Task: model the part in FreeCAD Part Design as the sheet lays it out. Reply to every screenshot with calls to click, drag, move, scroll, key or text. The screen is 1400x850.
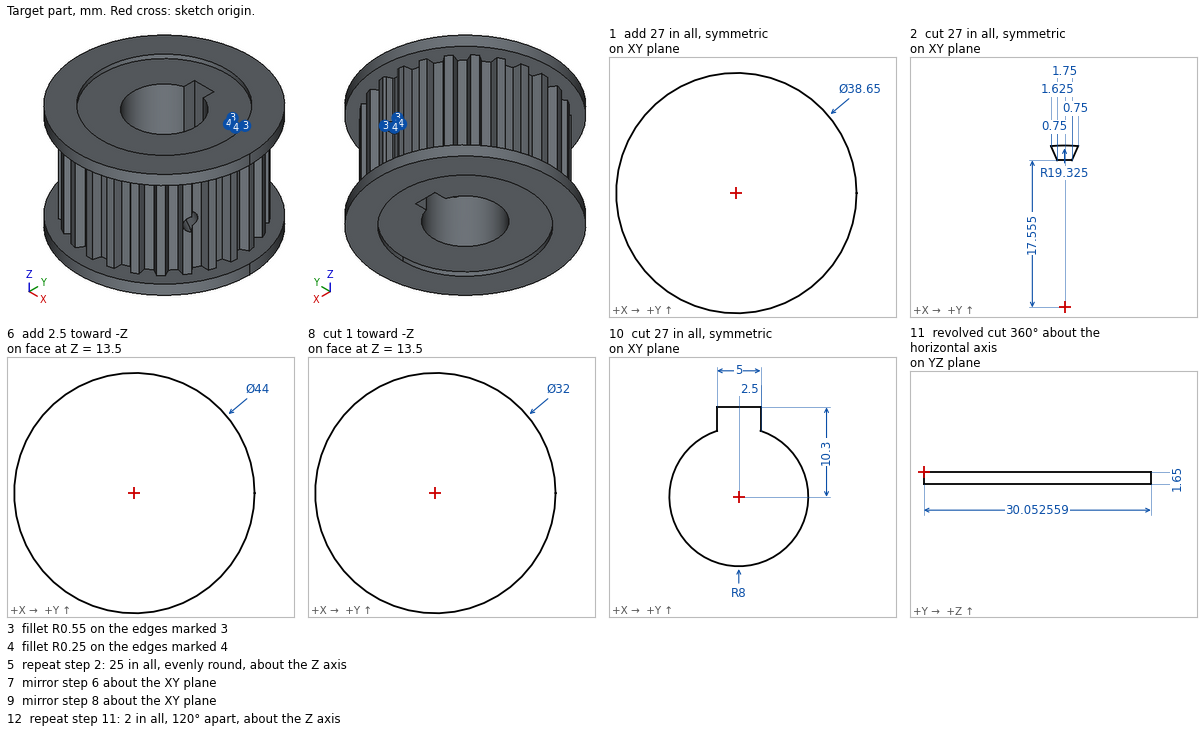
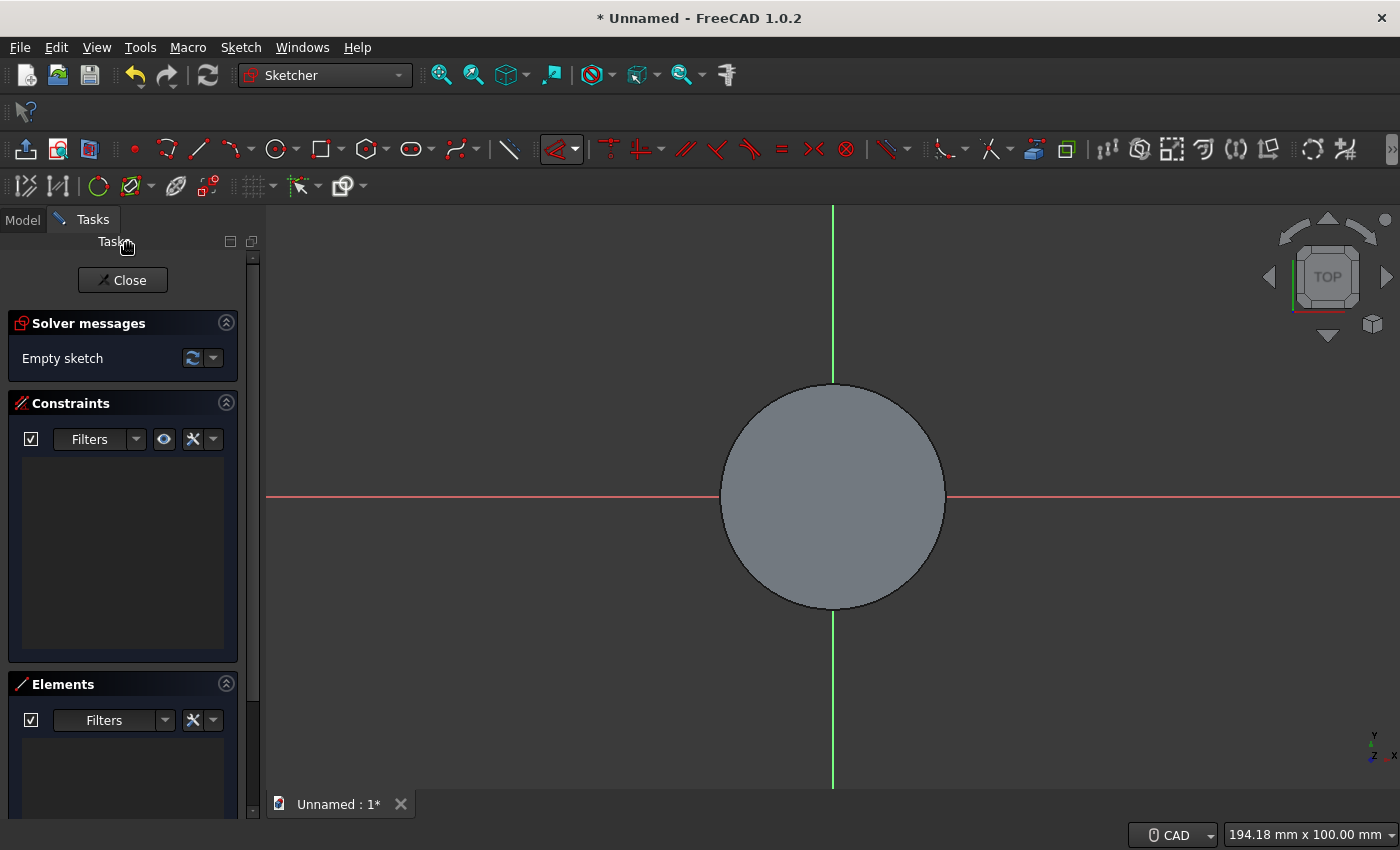
click(90, 150)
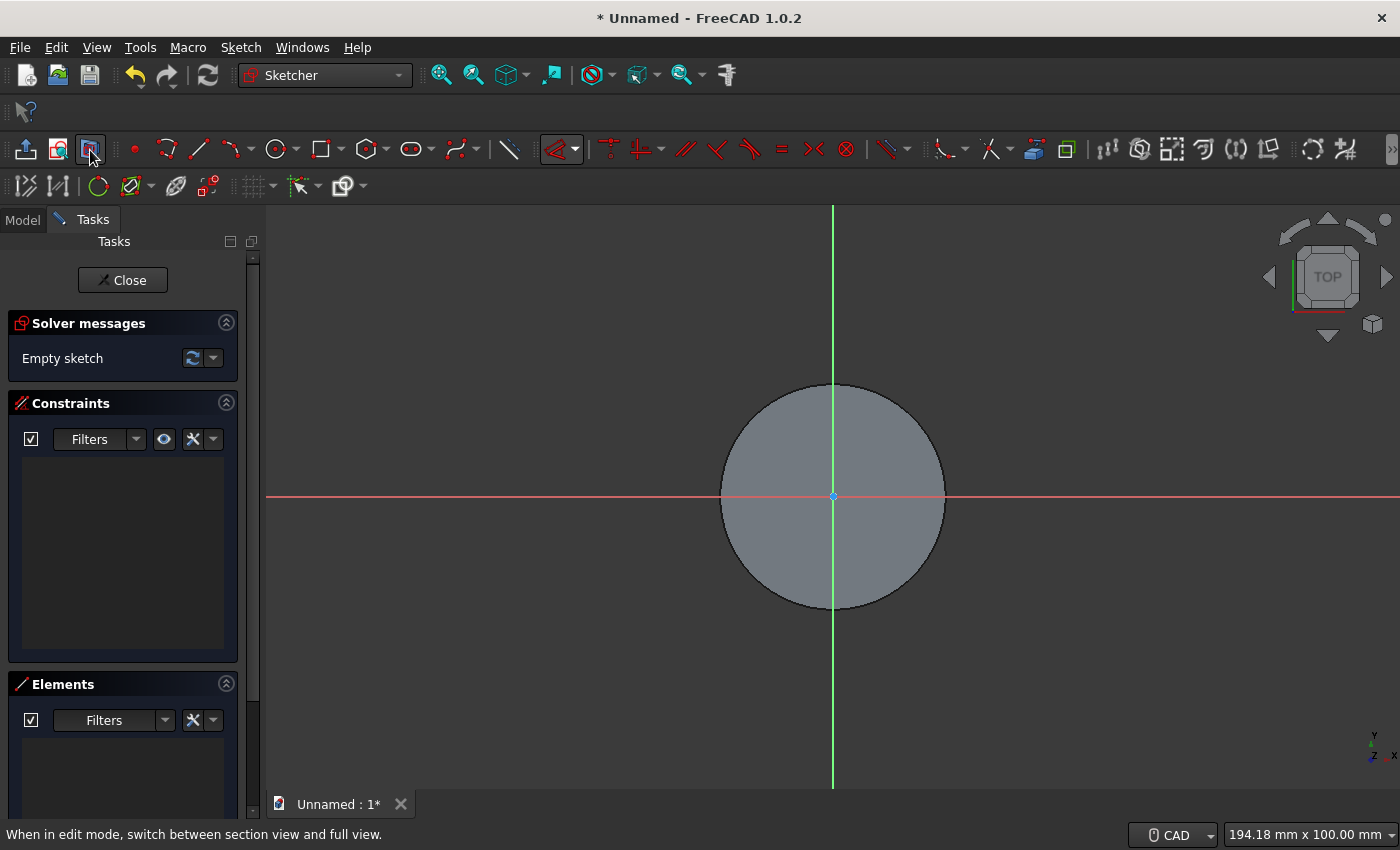
scroll(837, 384, up, 15)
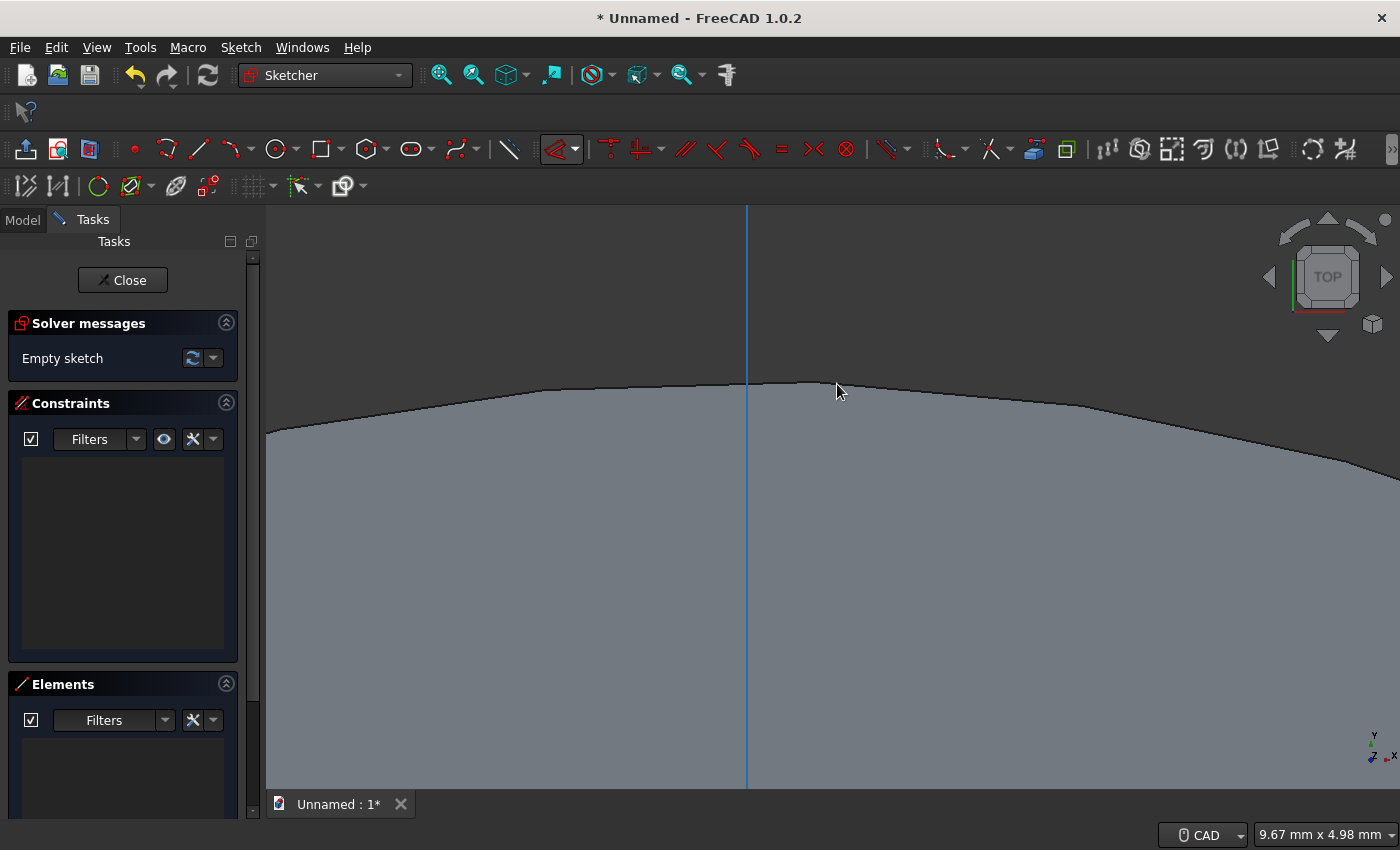
scroll(726, 470, up, 3)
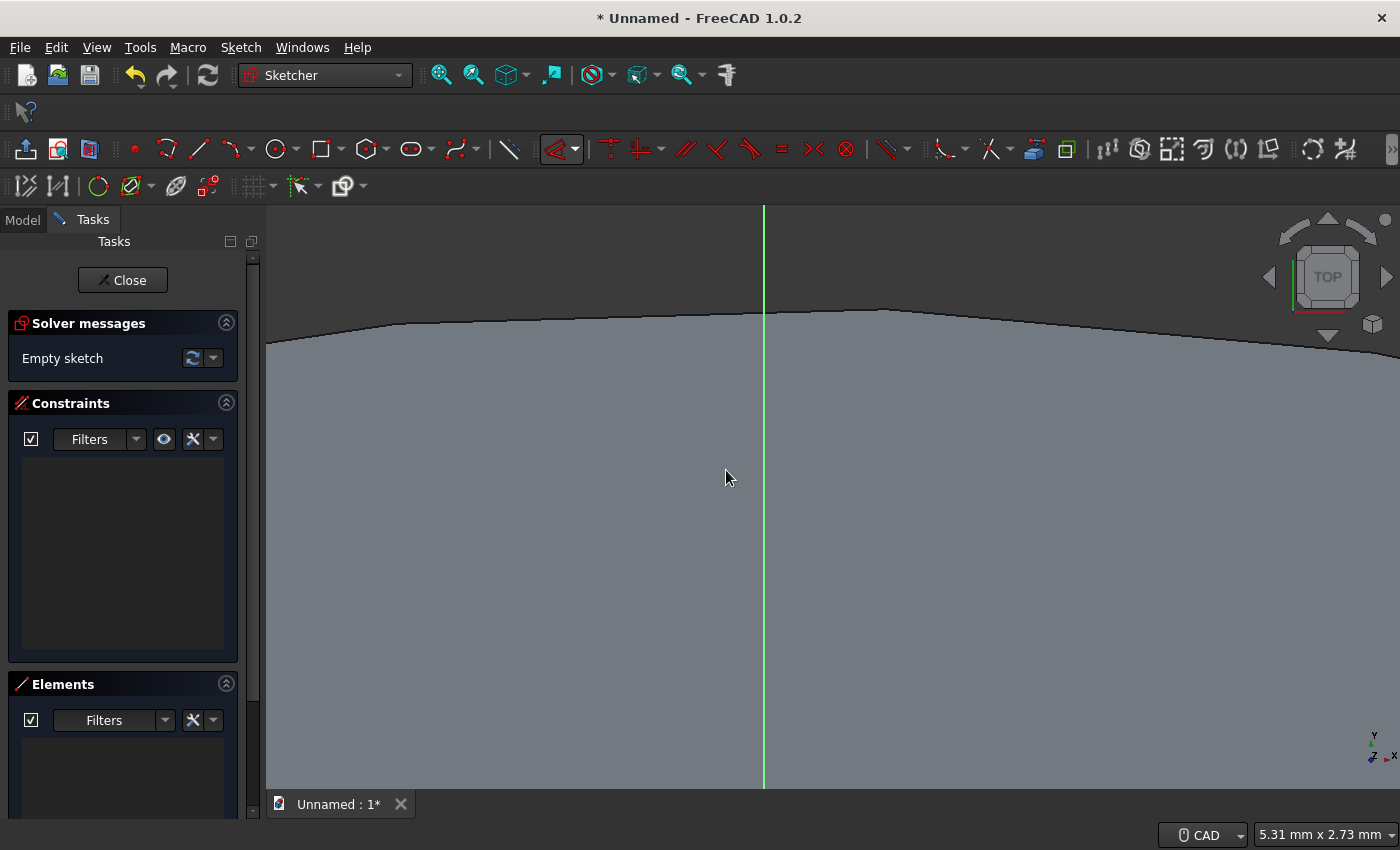
click(168, 150)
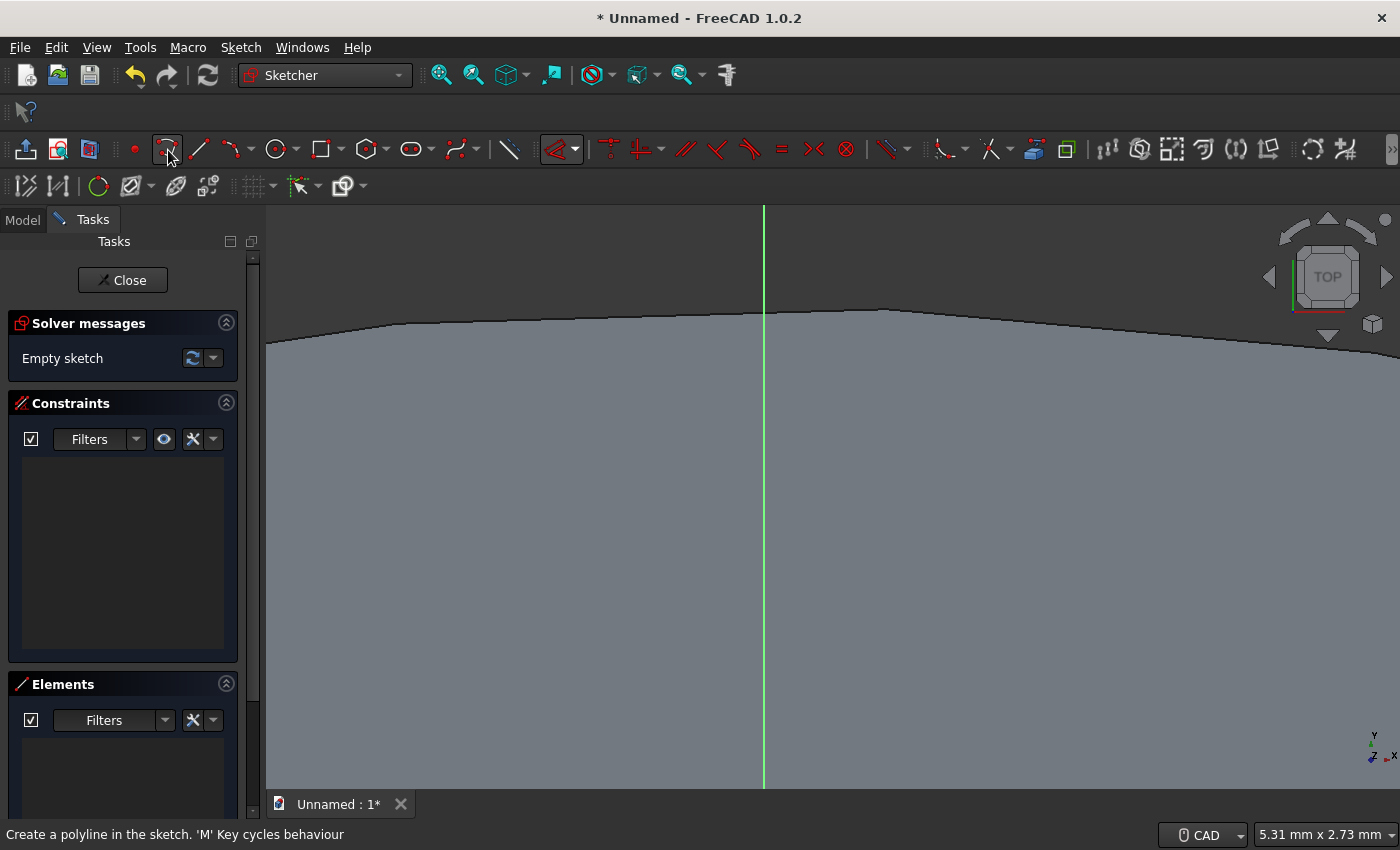
click(417, 322)
click(577, 686)
click(951, 686)
click(1111, 322)
right_click(1111, 322)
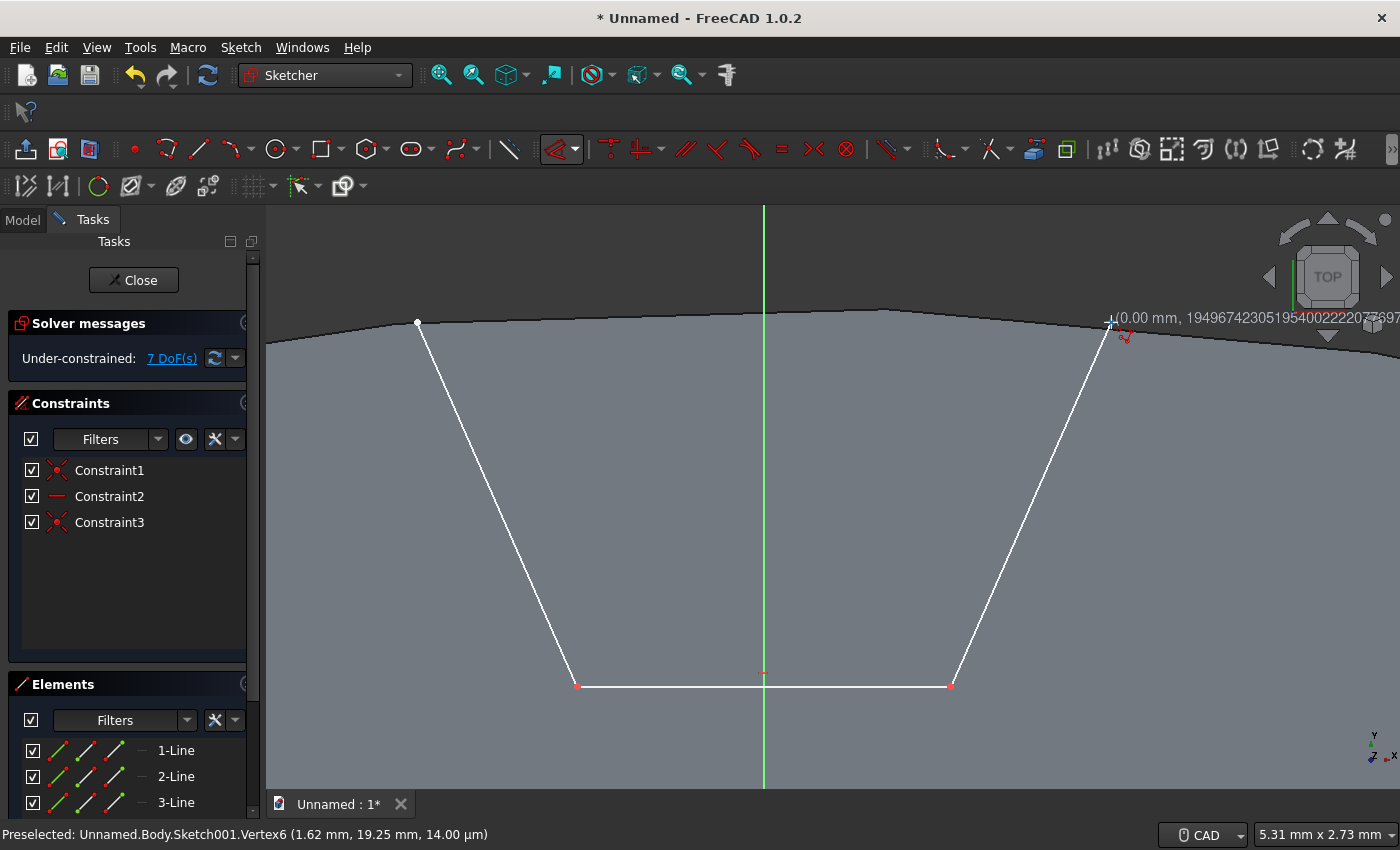
click(232, 150)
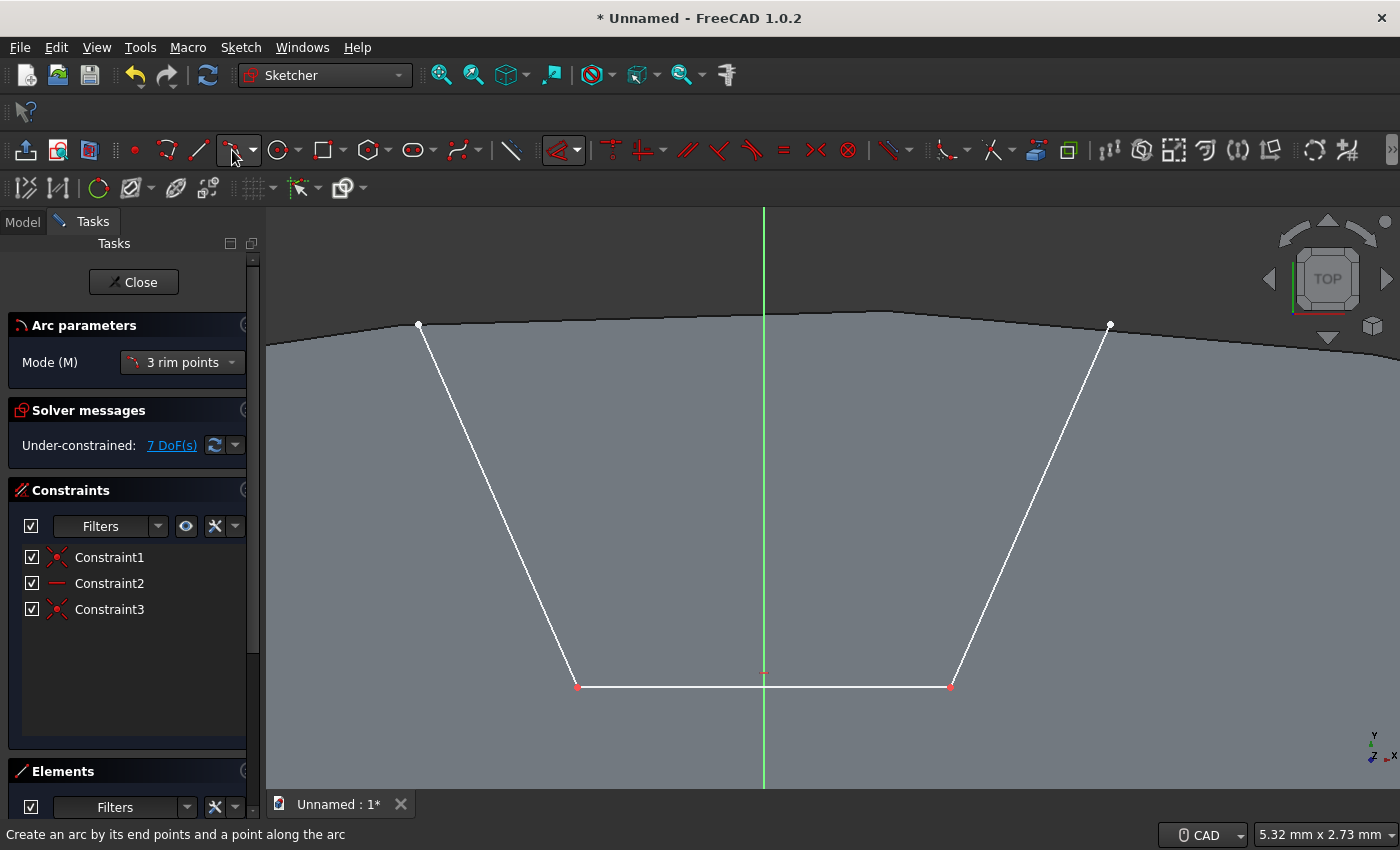
click(1110, 325)
click(418, 325)
click(834, 310)
key(Escape)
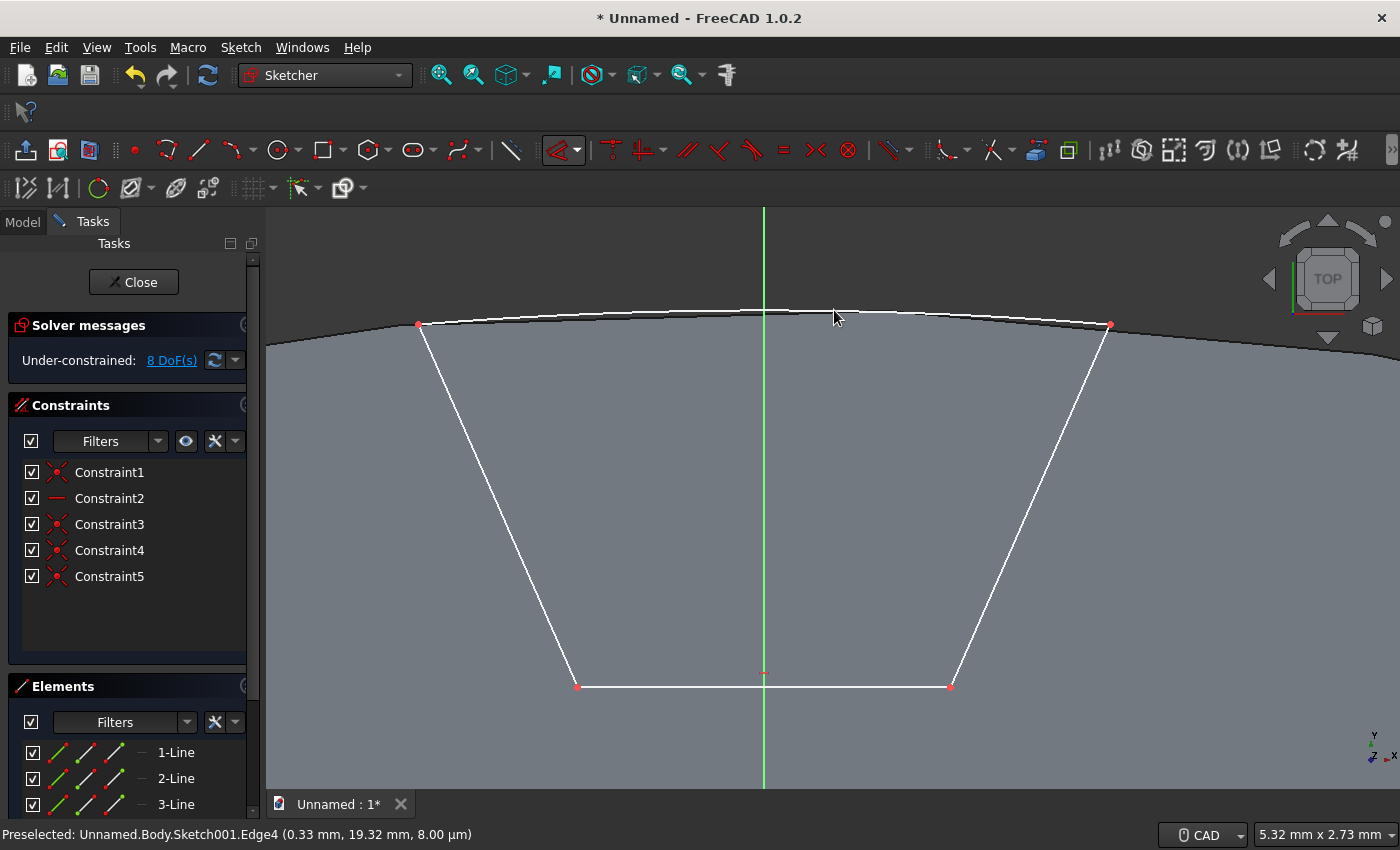
scroll(765, 309, down, 12)